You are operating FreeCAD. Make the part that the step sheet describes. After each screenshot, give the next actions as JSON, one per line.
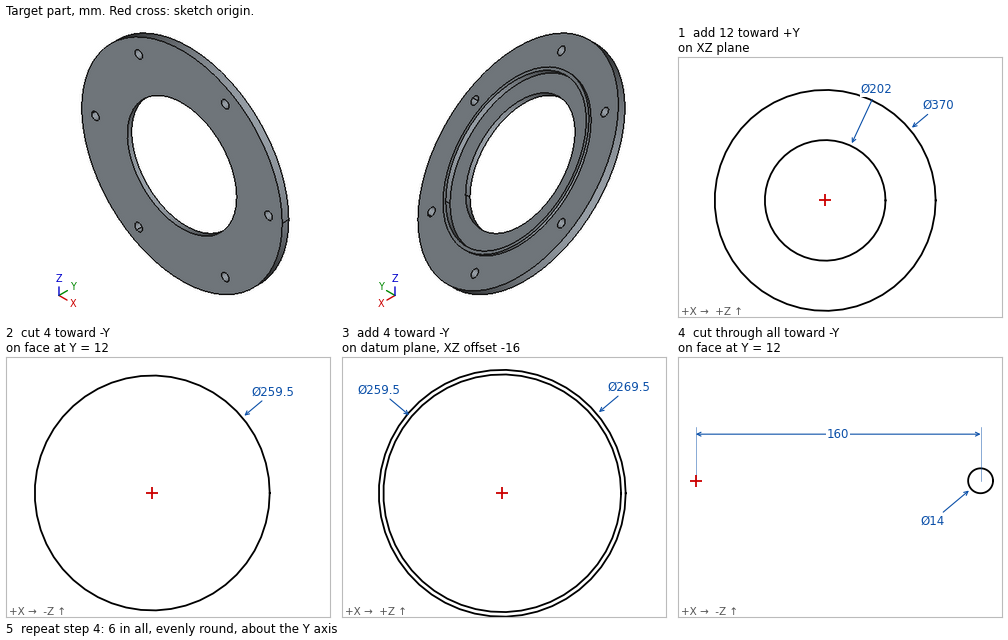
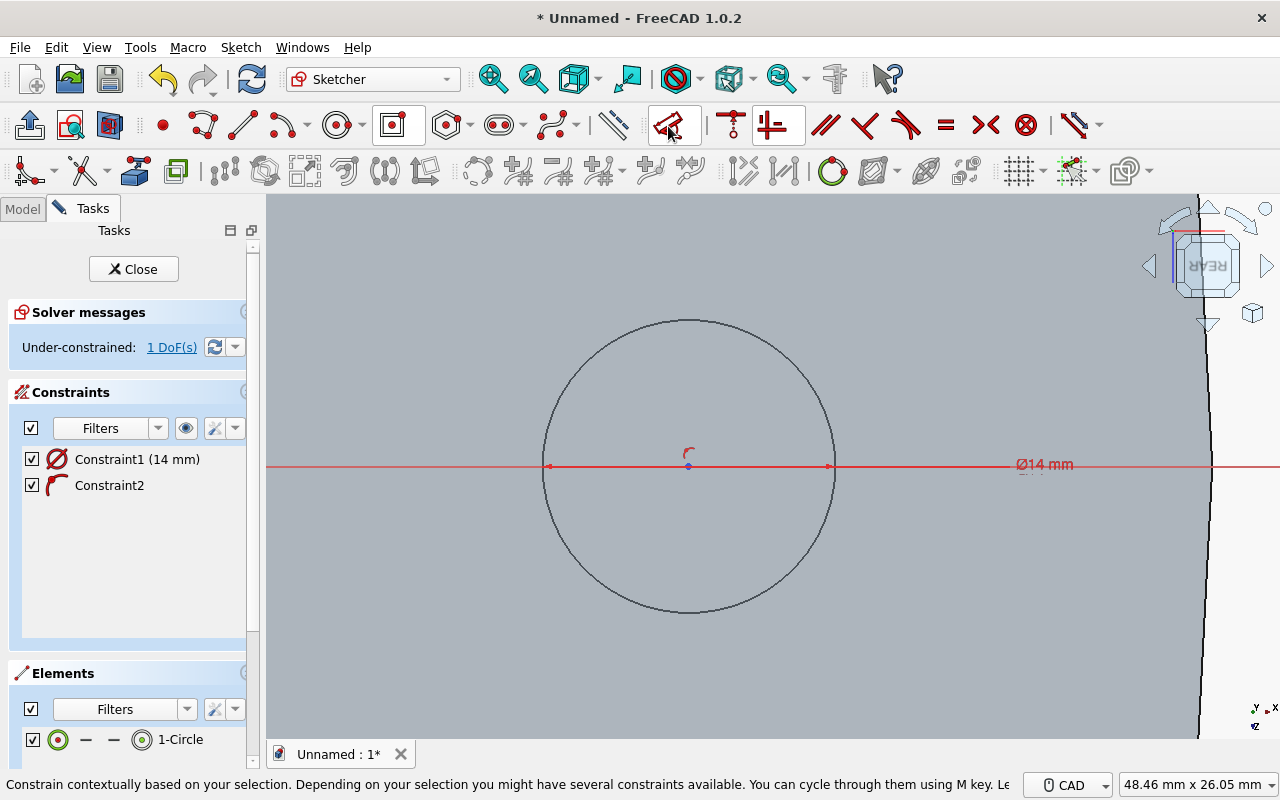
{"action": "left_click", "coordinate": [689, 466]}
{"action": "left_click", "coordinate": [491, 500]}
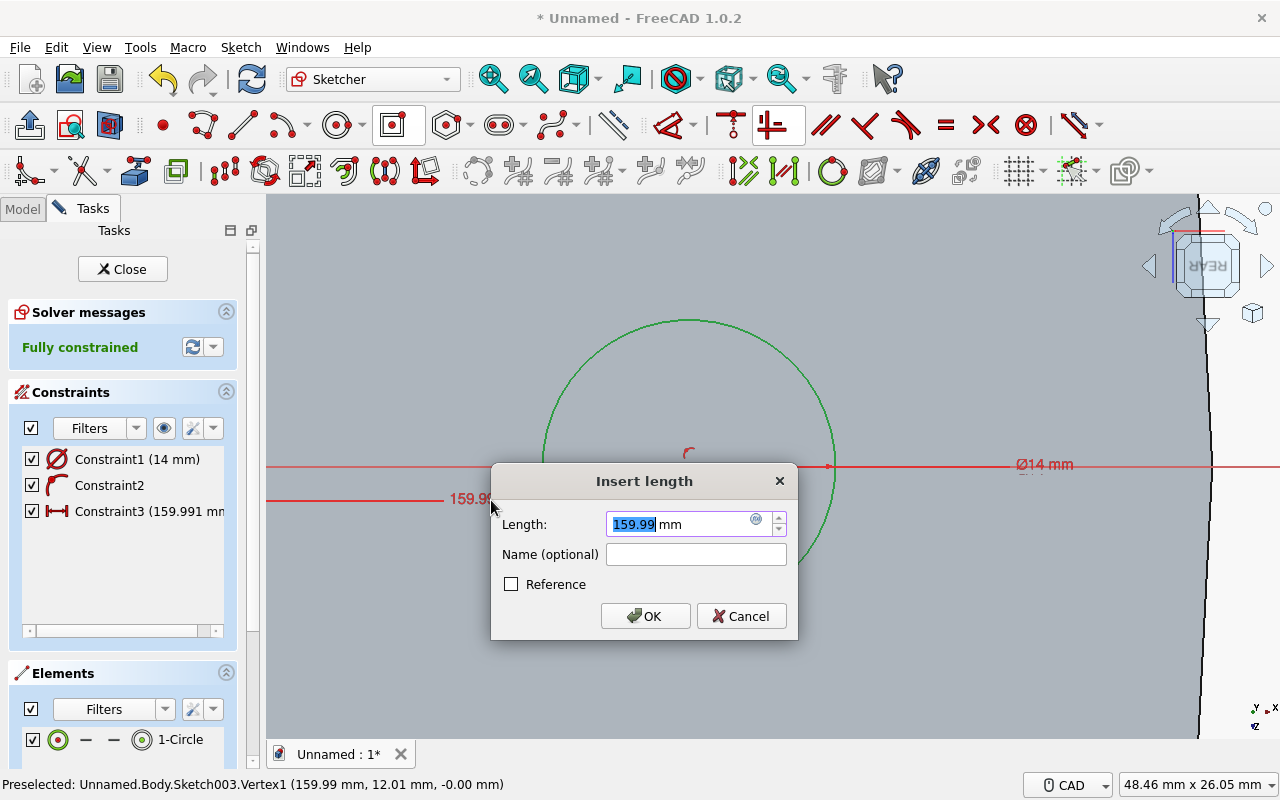
{"action": "type", "text": "160"}
{"action": "key", "text": "Return"}
{"action": "key", "text": "Escape"}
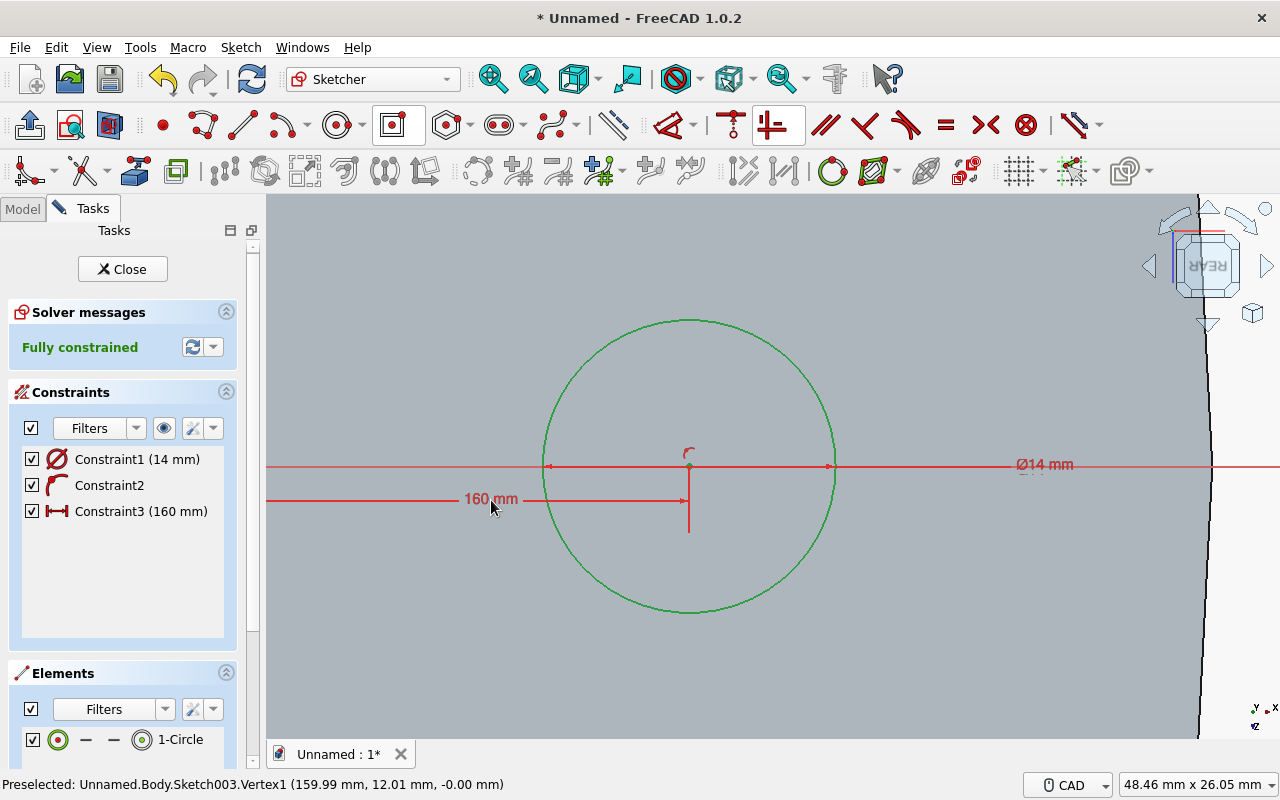
{"action": "left_click", "coordinate": [123, 269]}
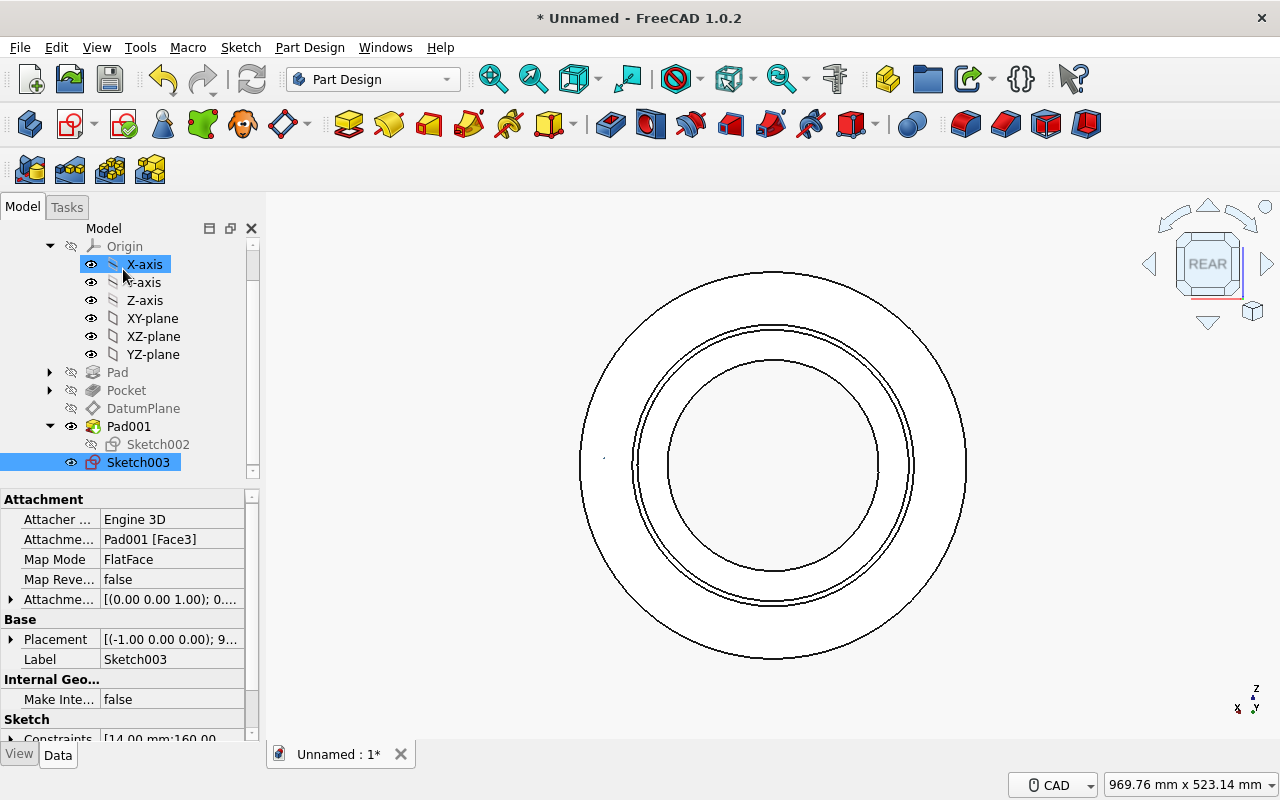
{"action": "left_click", "coordinate": [612, 124]}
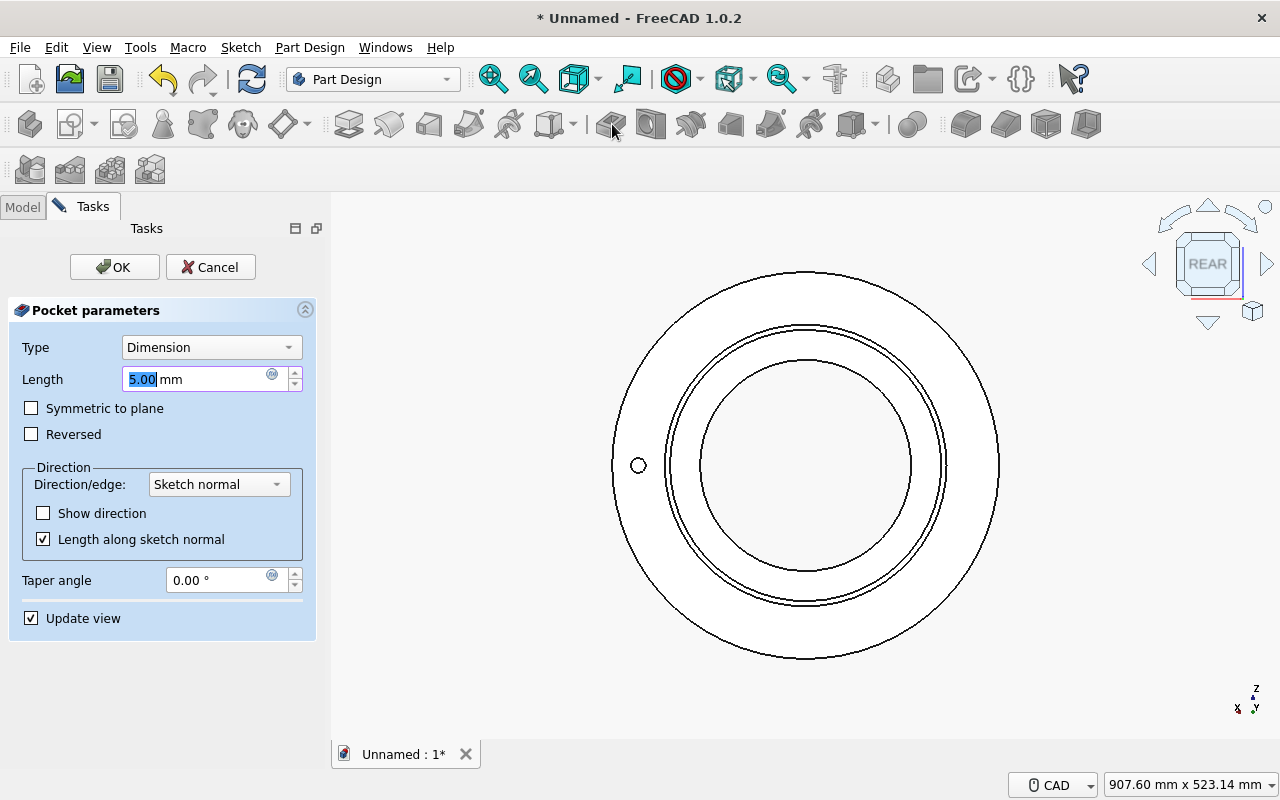
{"action": "left_click", "coordinate": [212, 348]}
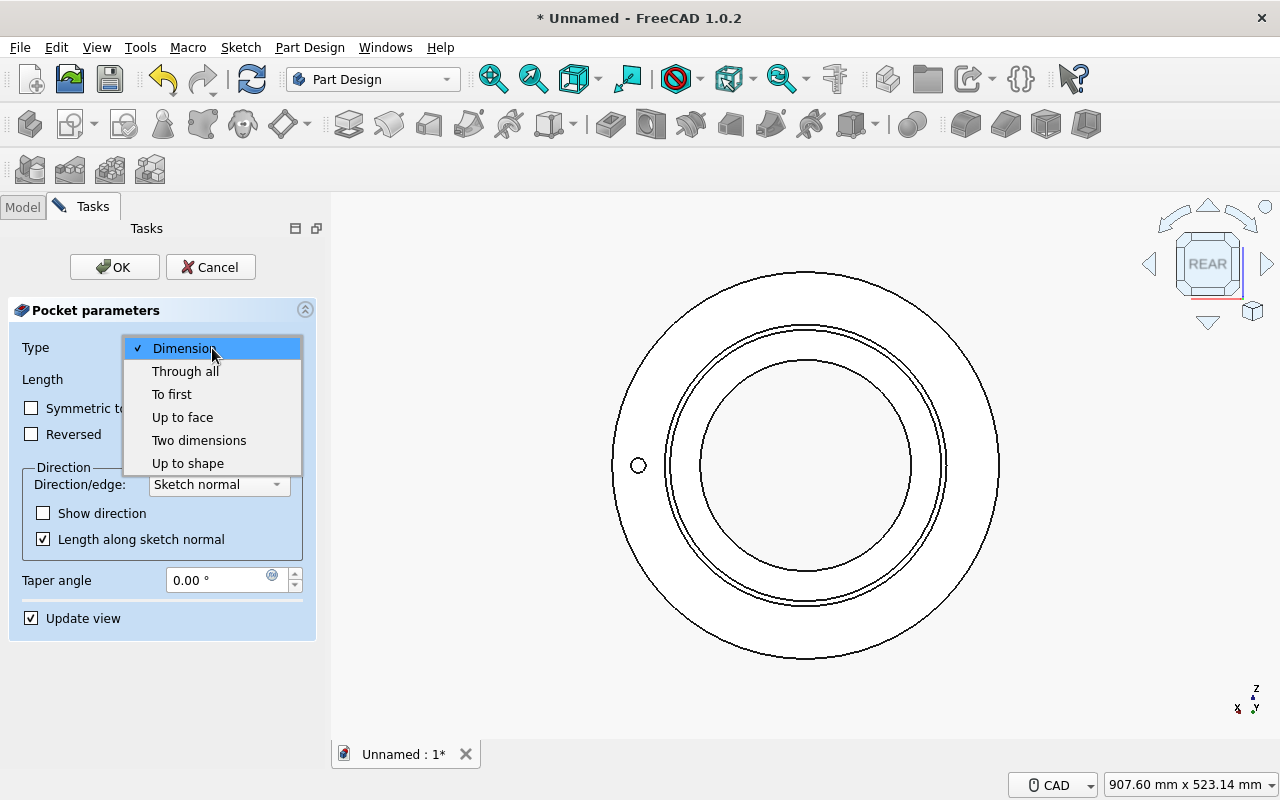
{"action": "left_click", "coordinate": [212, 372]}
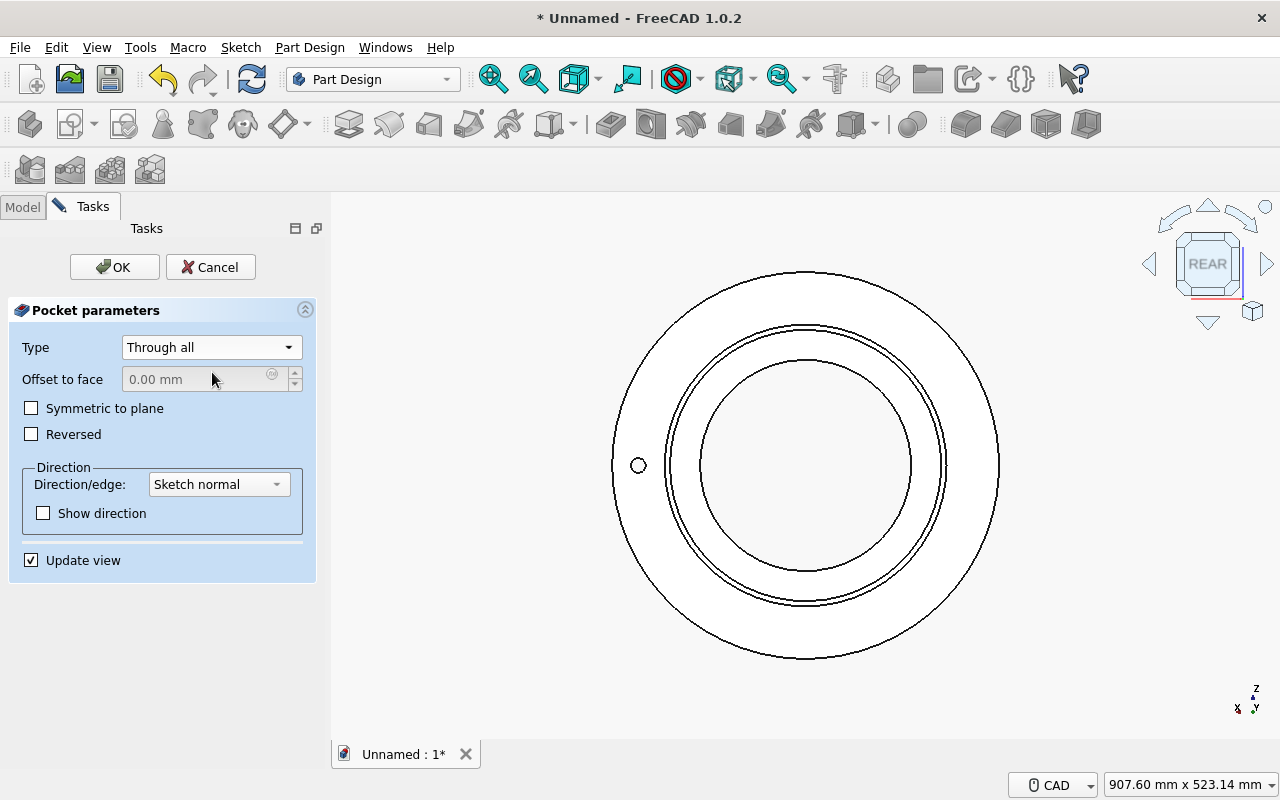
{"action": "left_click", "coordinate": [115, 267]}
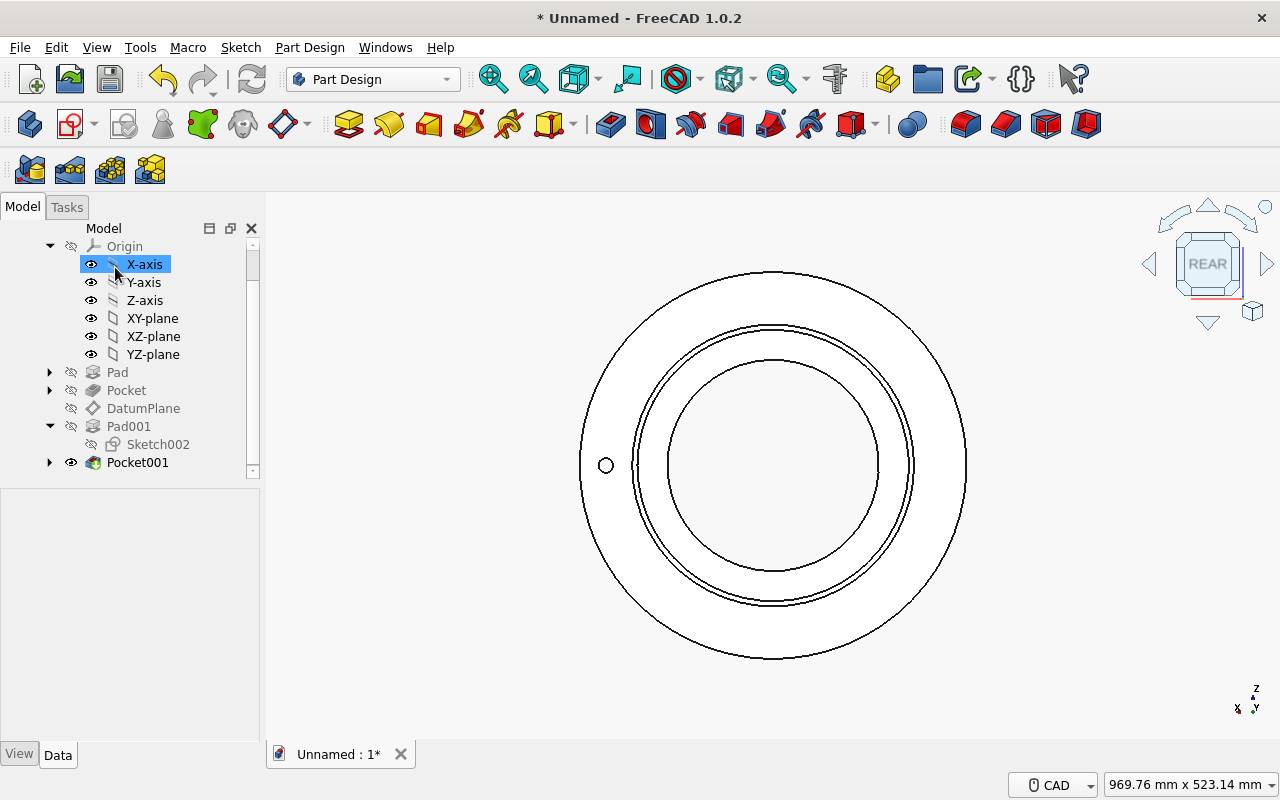
{"action": "left_click", "coordinate": [116, 462]}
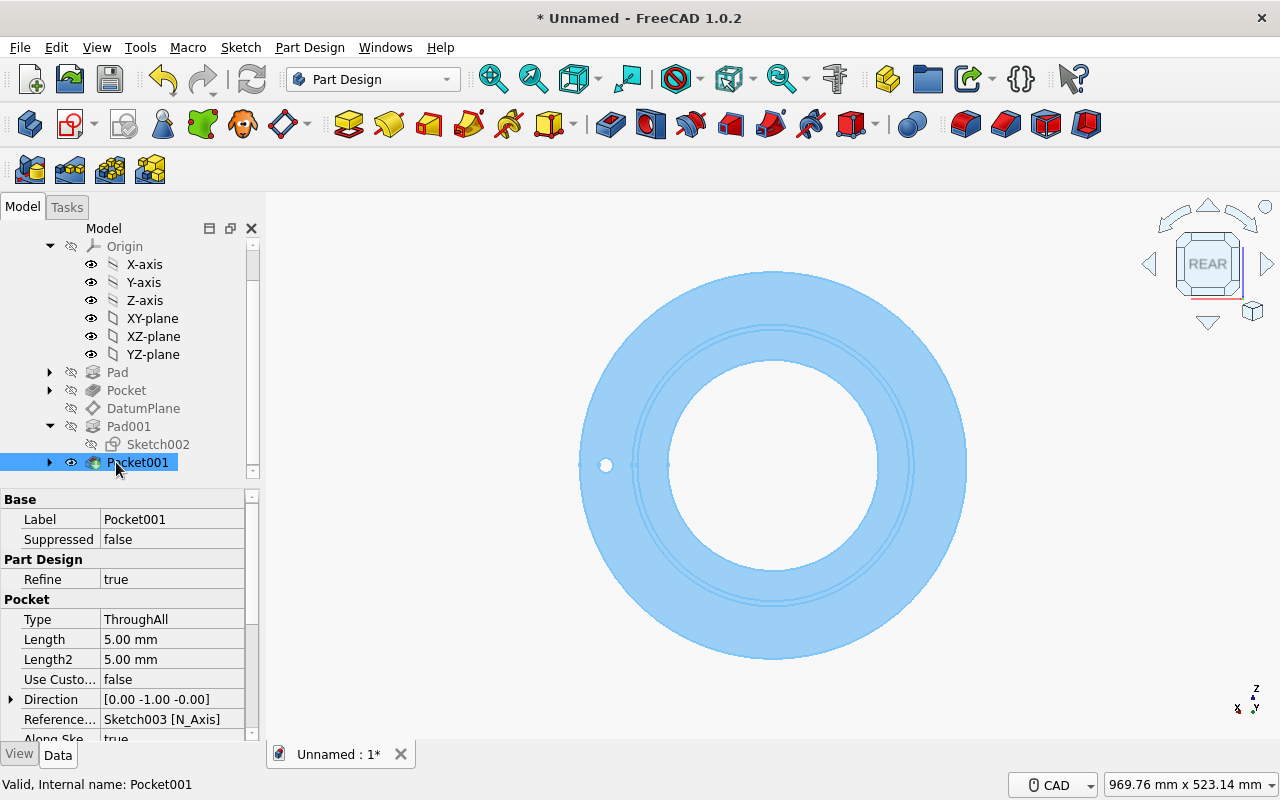
{"action": "left_click", "coordinate": [110, 170]}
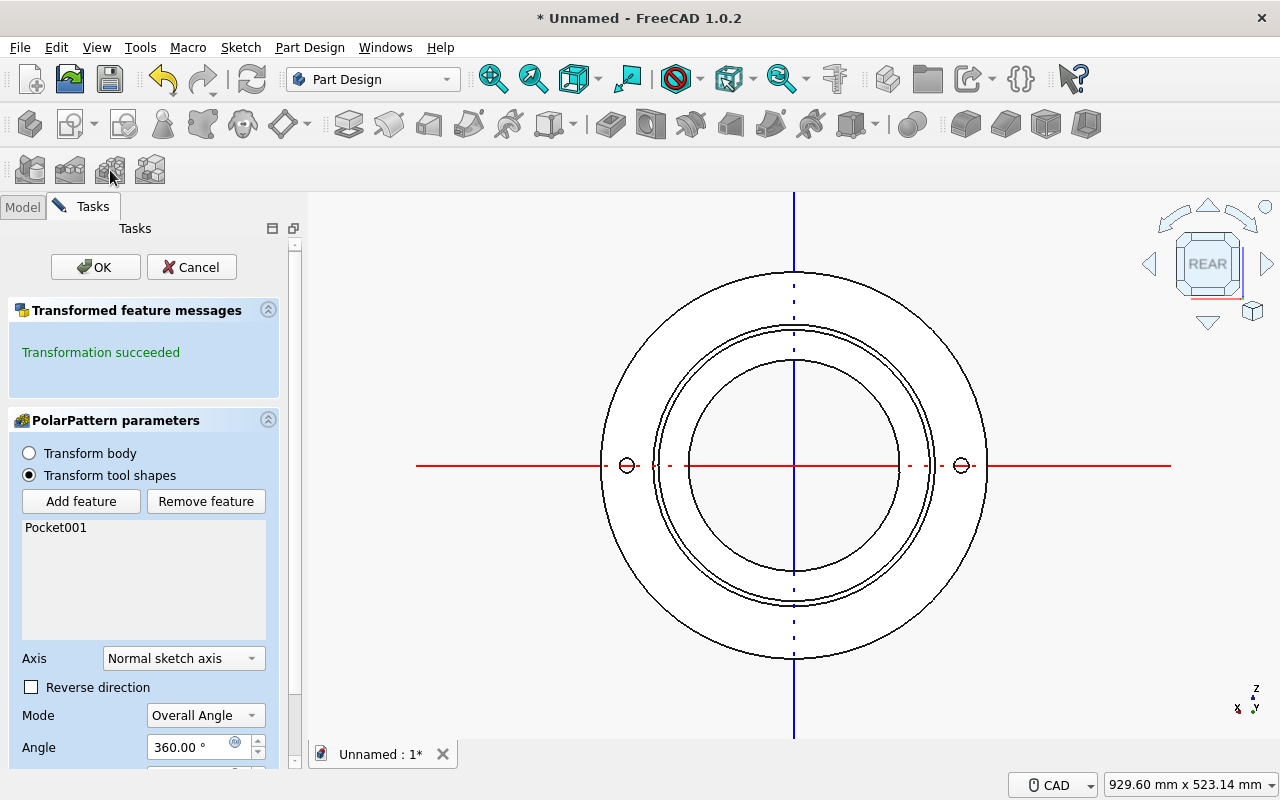
{"action": "left_click", "coordinate": [184, 658]}